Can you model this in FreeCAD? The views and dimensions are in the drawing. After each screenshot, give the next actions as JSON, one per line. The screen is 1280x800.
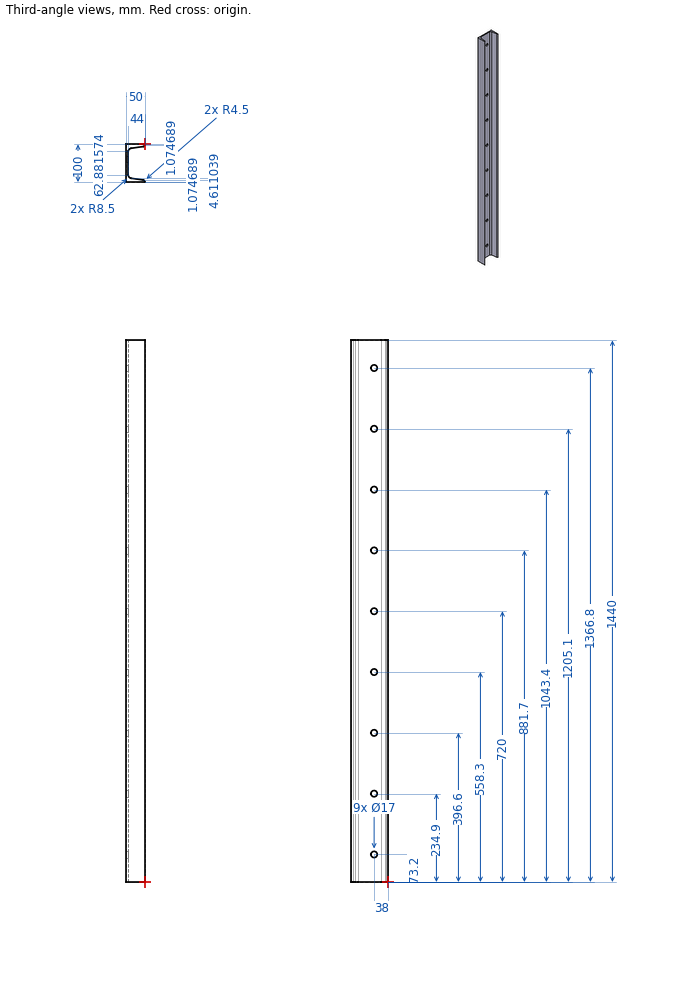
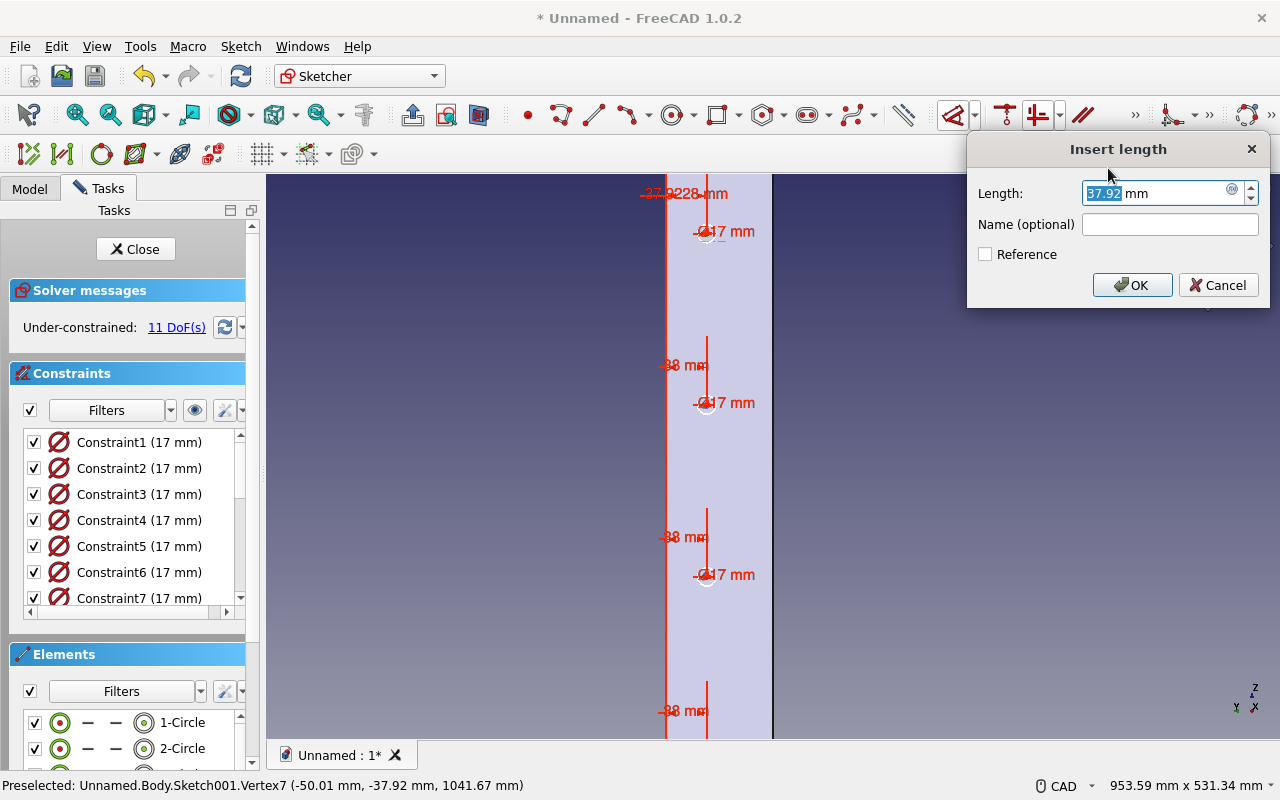
{"action": "type", "text": "38"}
{"action": "key", "text": "Return"}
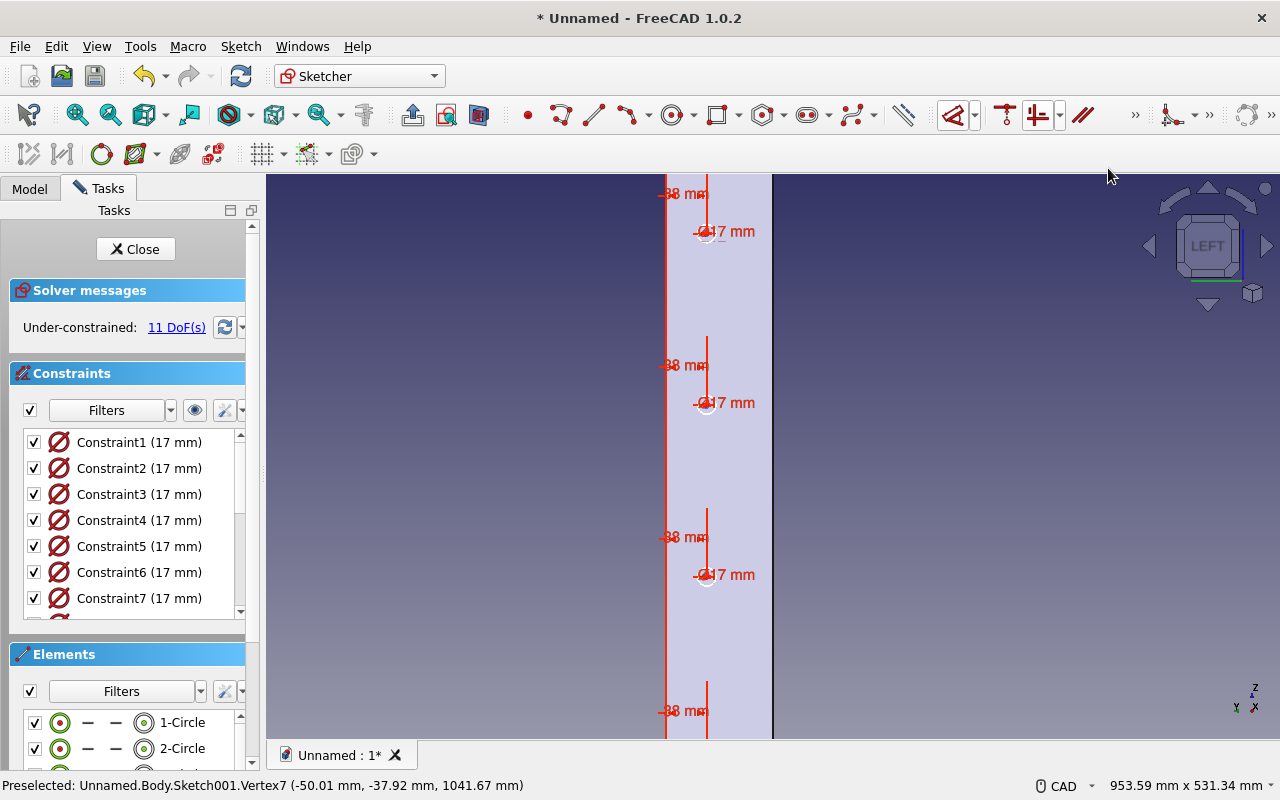
{"action": "scroll", "coordinate": [709, 406], "scroll_direction": "down", "scroll_amount": 7}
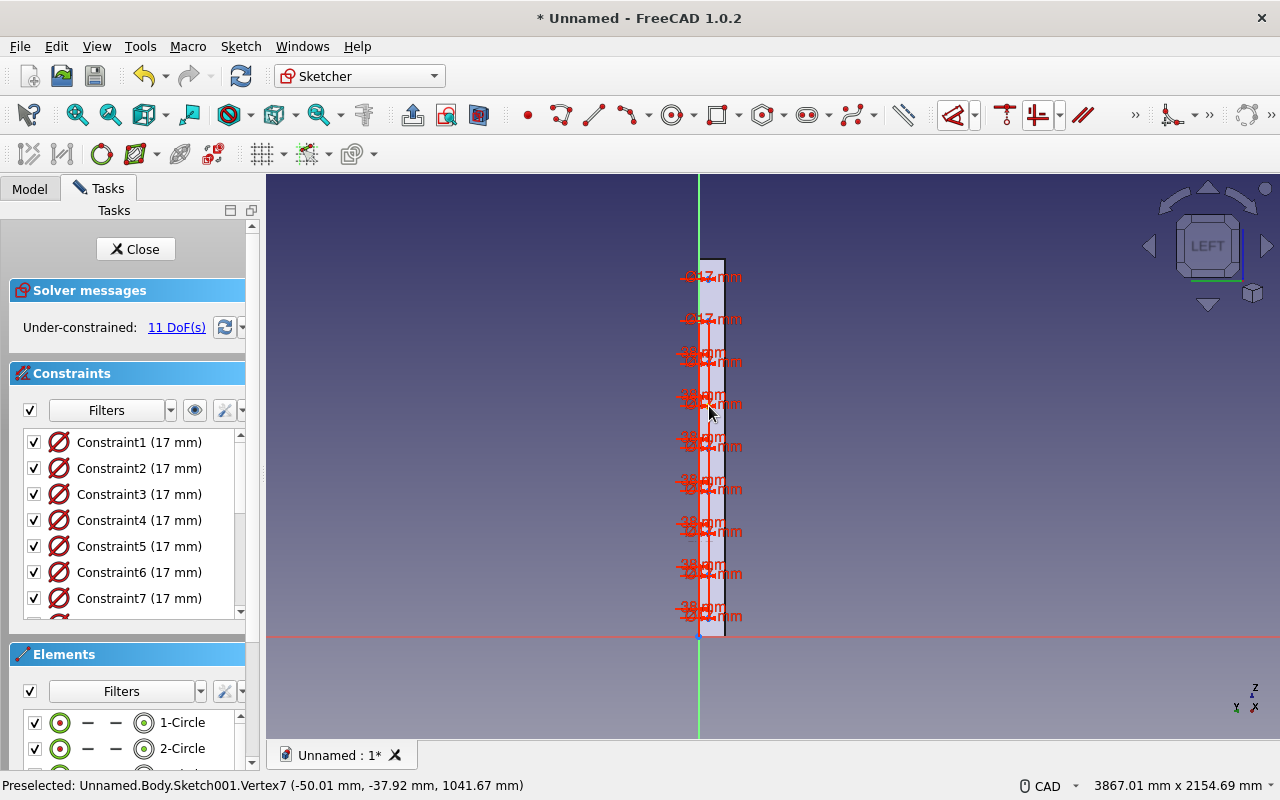
{"action": "scroll", "coordinate": [709, 321], "scroll_direction": "up", "scroll_amount": 7}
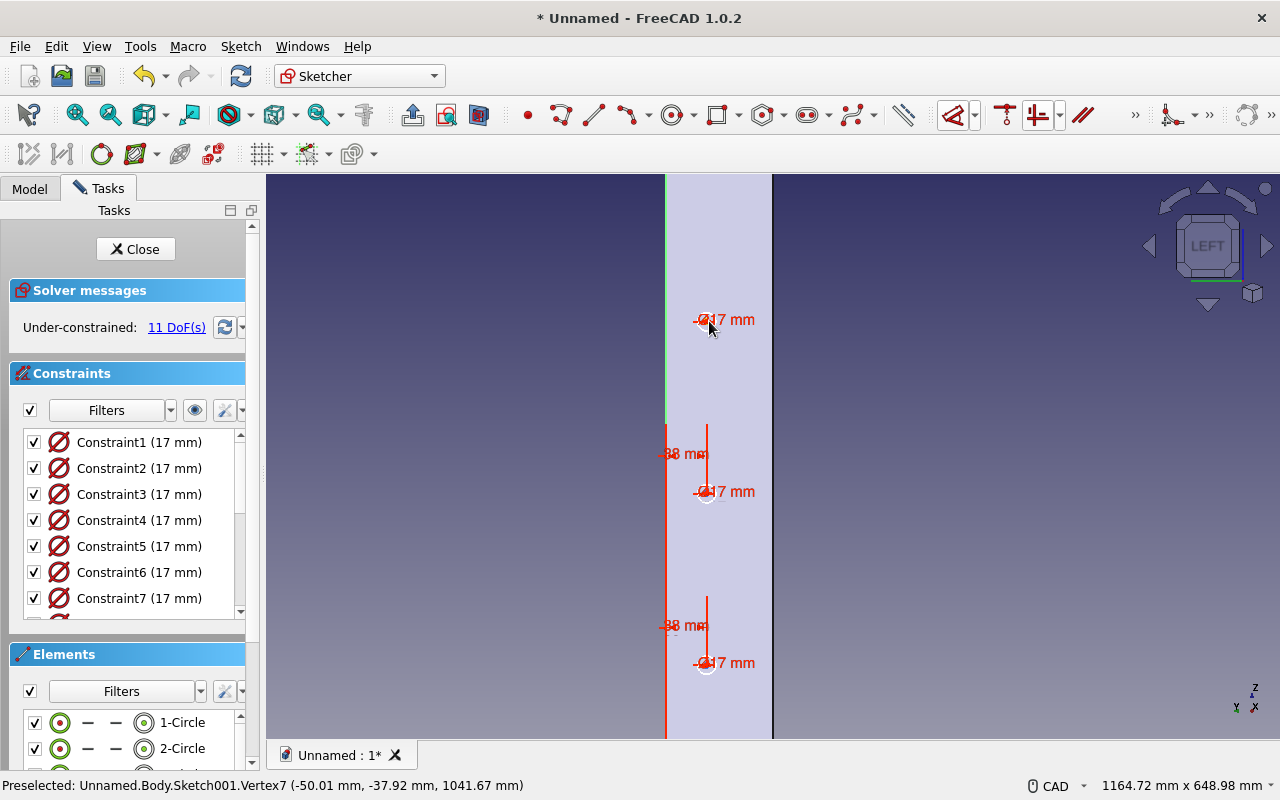
{"action": "left_click", "coordinate": [707, 322]}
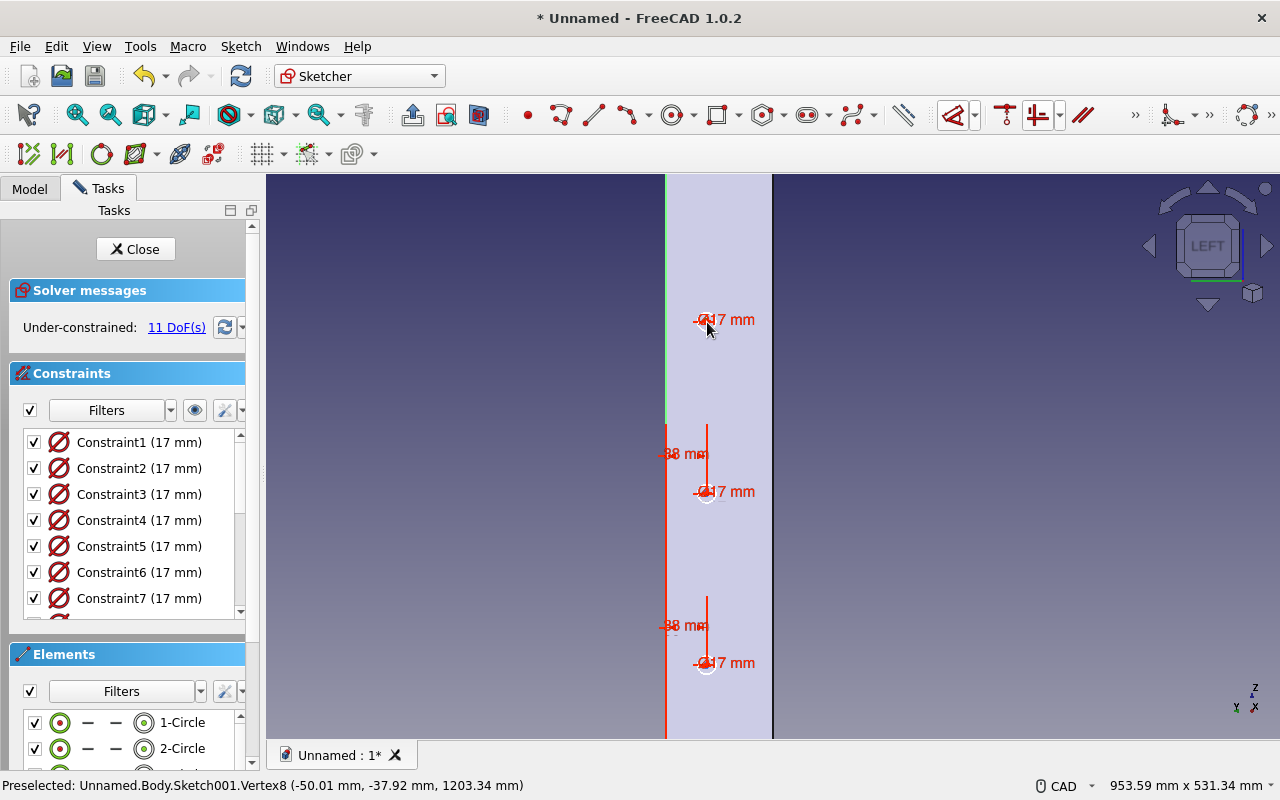
{"action": "key", "text": "l"}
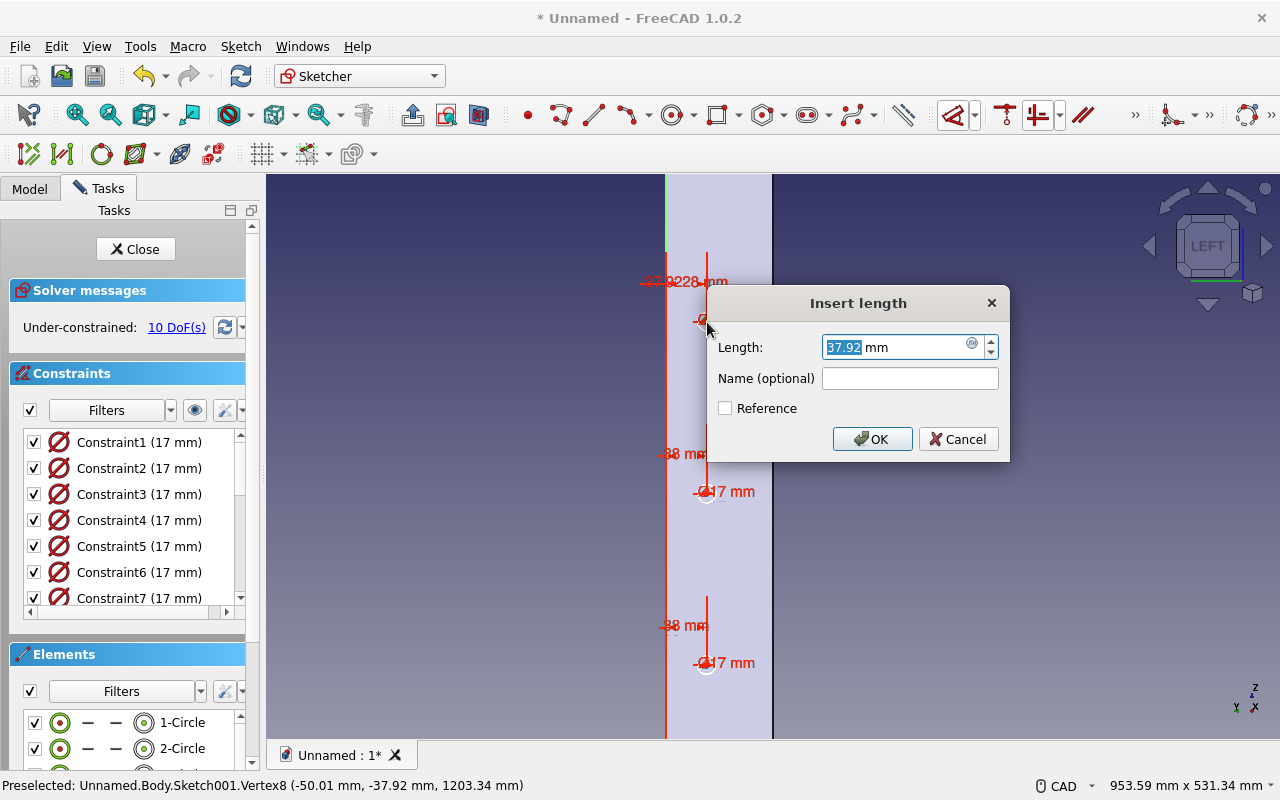
{"action": "type", "text": "38"}
{"action": "key", "text": "Return"}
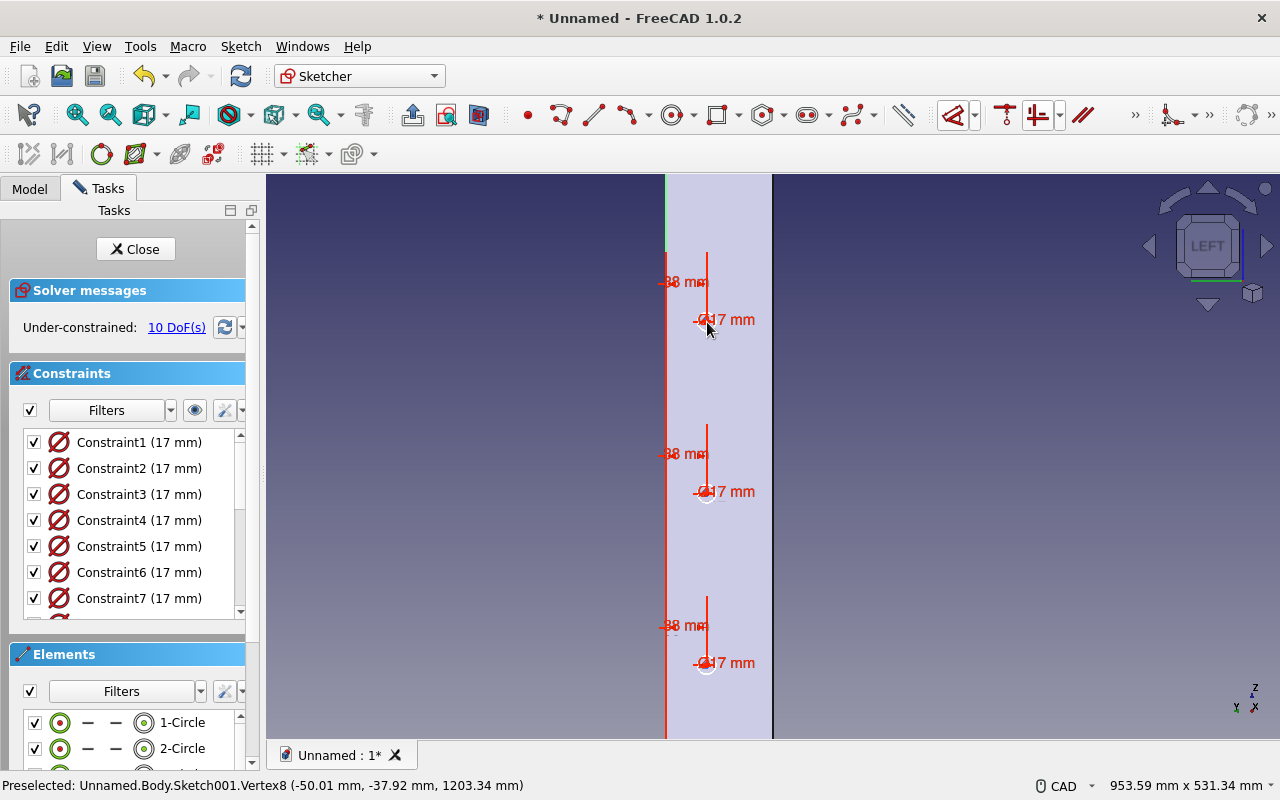
{"action": "scroll", "coordinate": [709, 321], "scroll_direction": "down", "scroll_amount": 7}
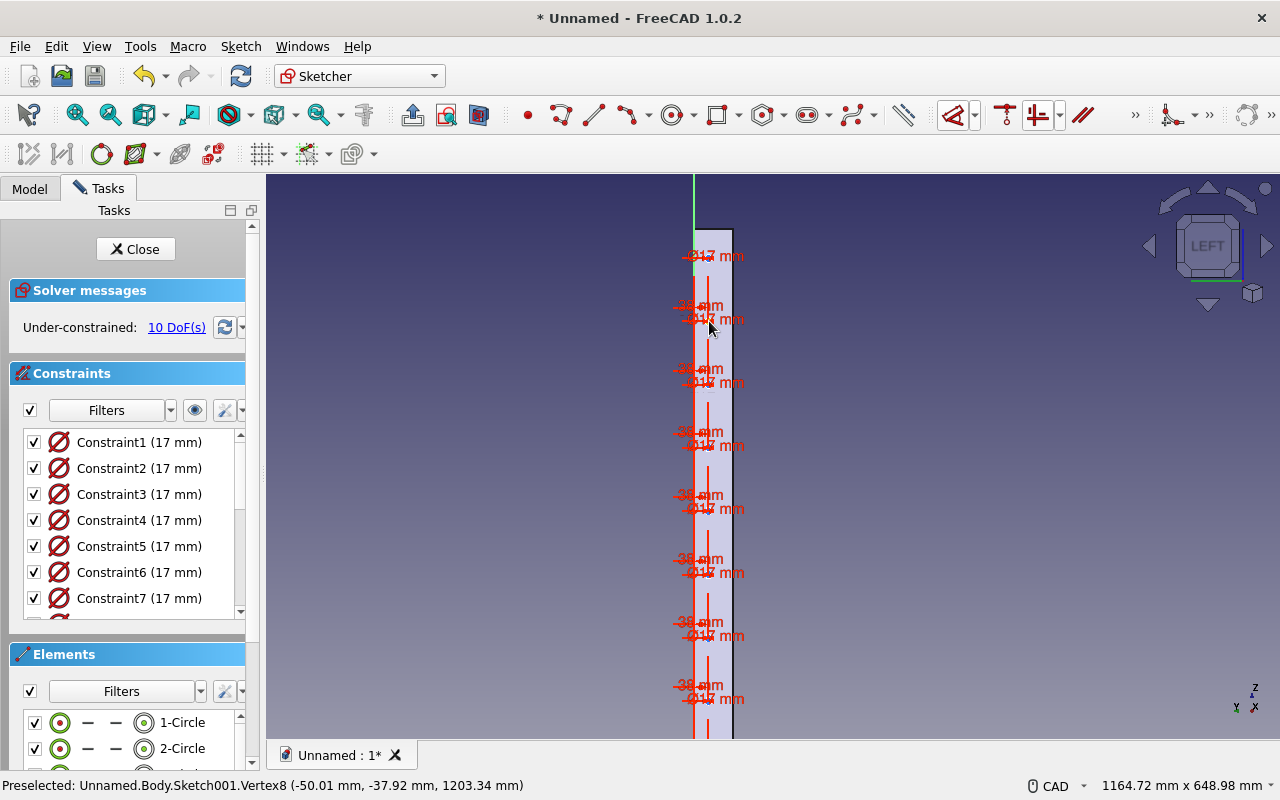
{"action": "scroll", "coordinate": [709, 279], "scroll_direction": "up", "scroll_amount": 7}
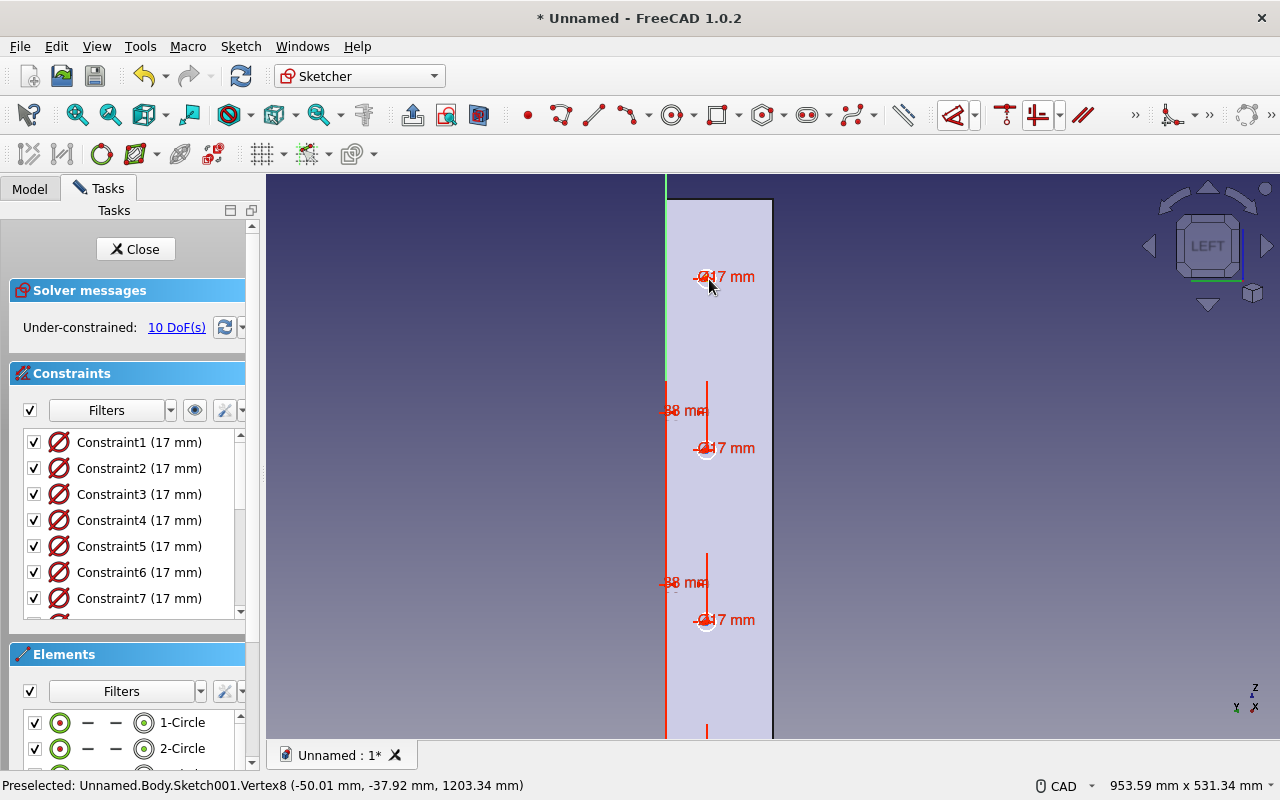
{"action": "left_click", "coordinate": [707, 279]}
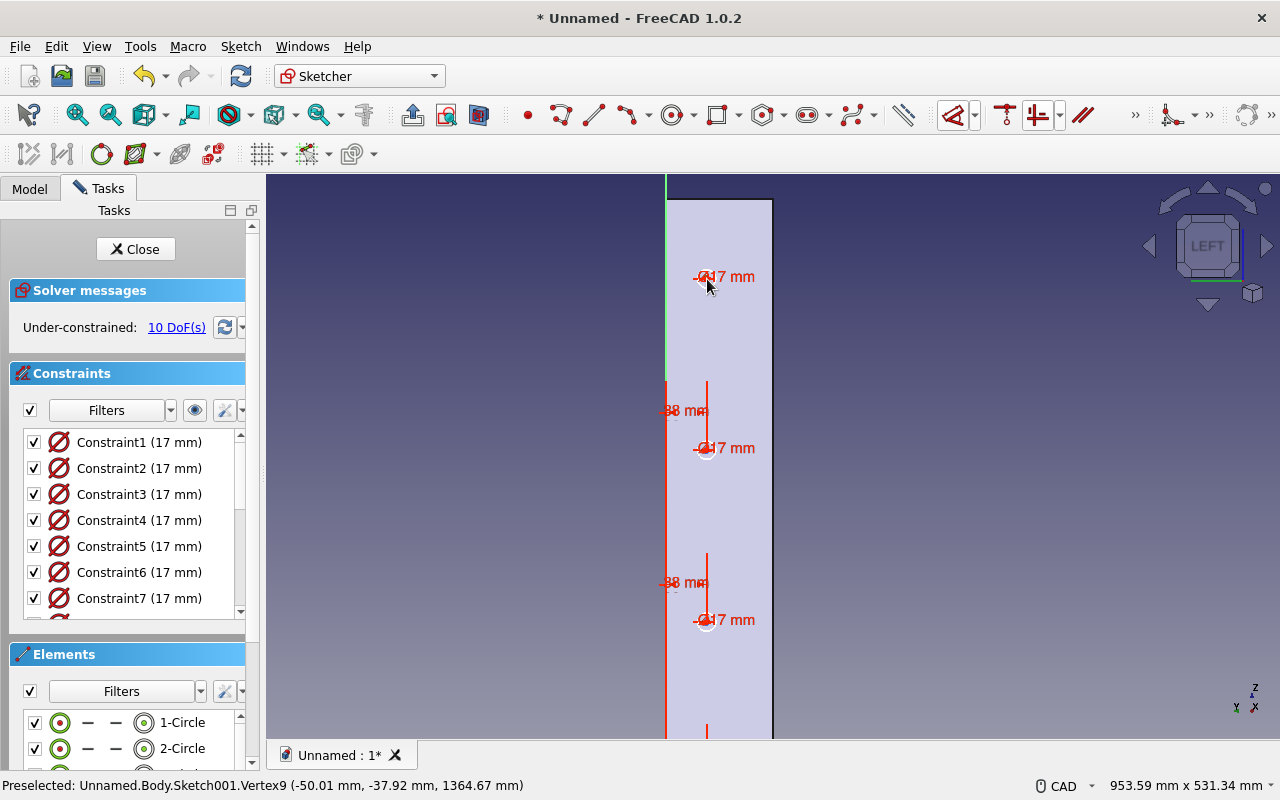
{"action": "left_click", "coordinate": [974, 116]}